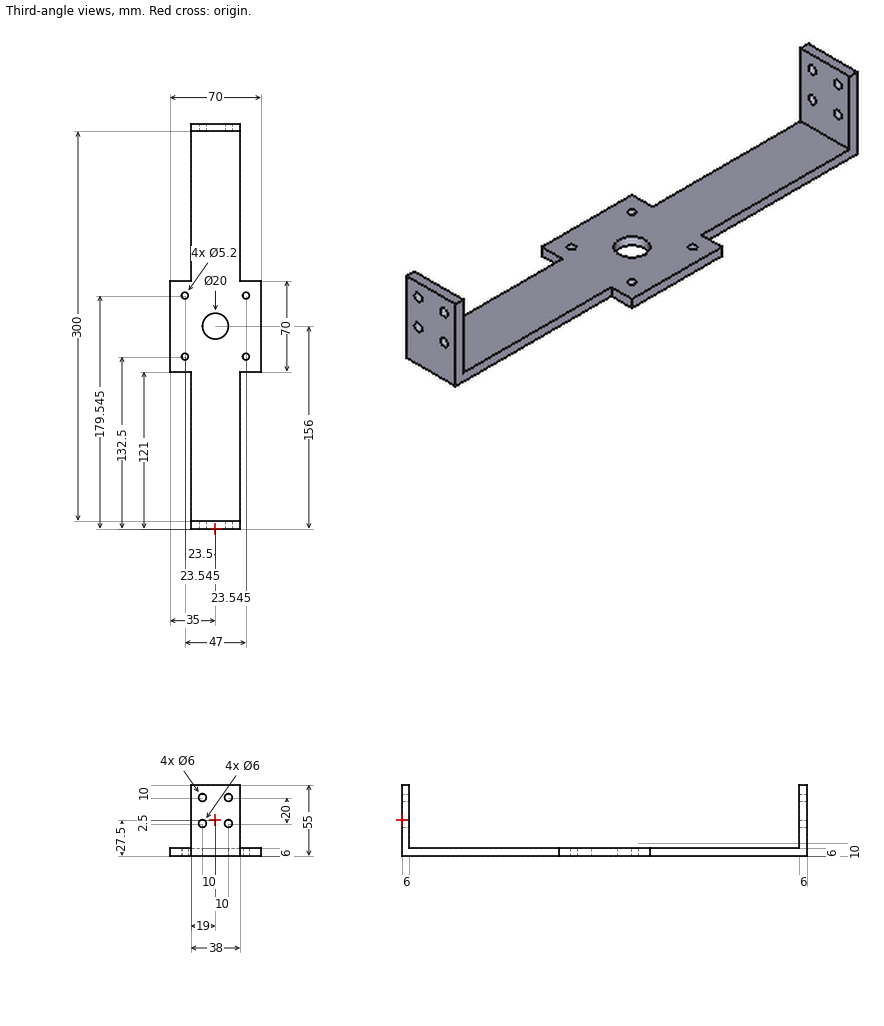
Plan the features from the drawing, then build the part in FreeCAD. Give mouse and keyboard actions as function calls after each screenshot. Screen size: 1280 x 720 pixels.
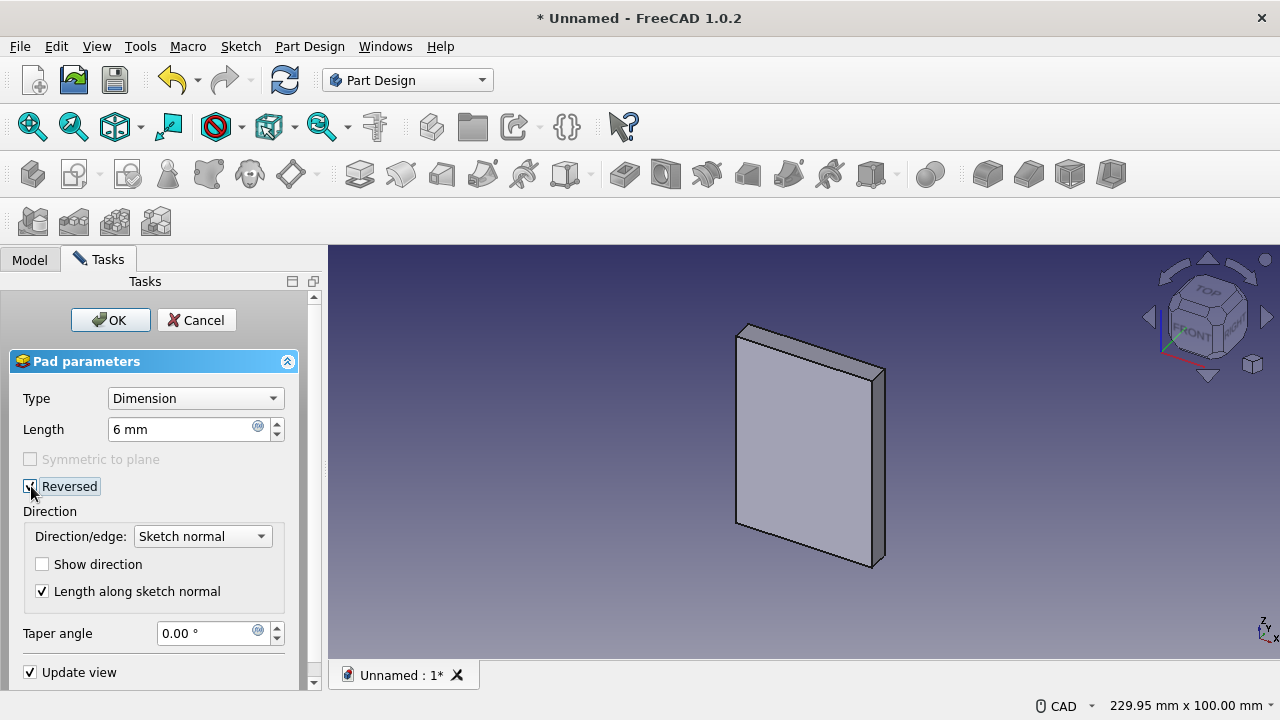
click(111, 320)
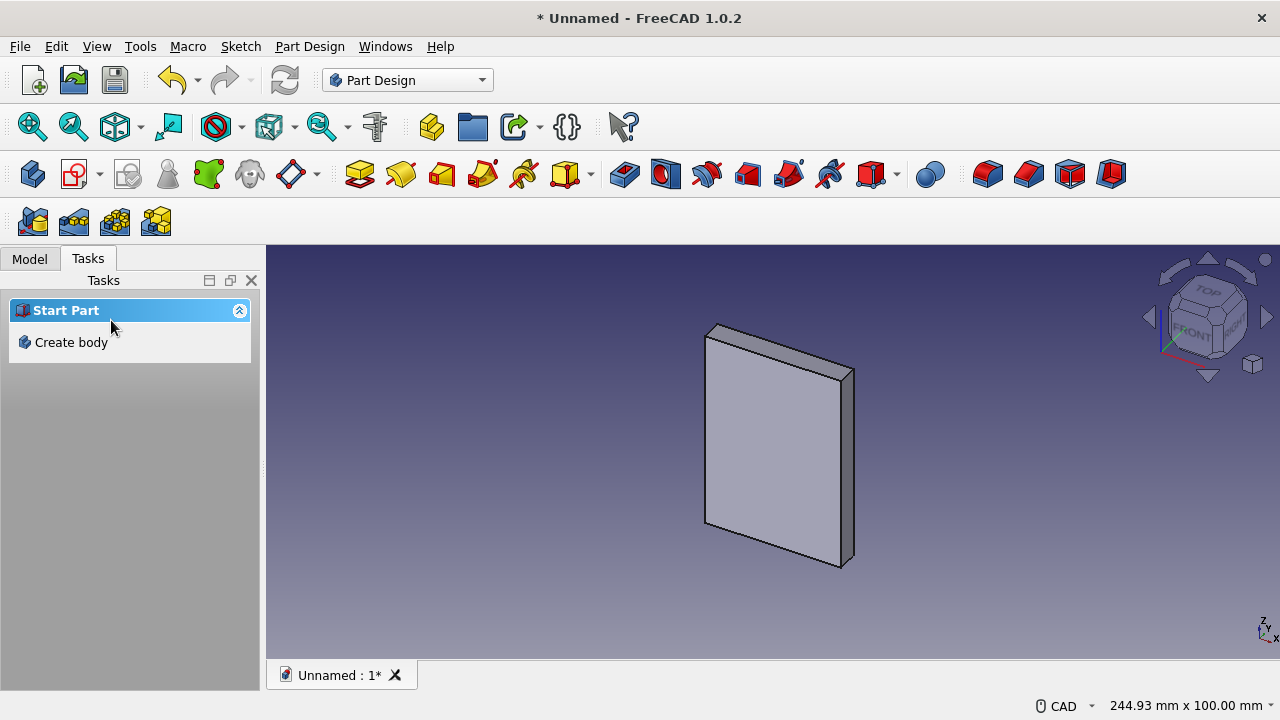
key(4)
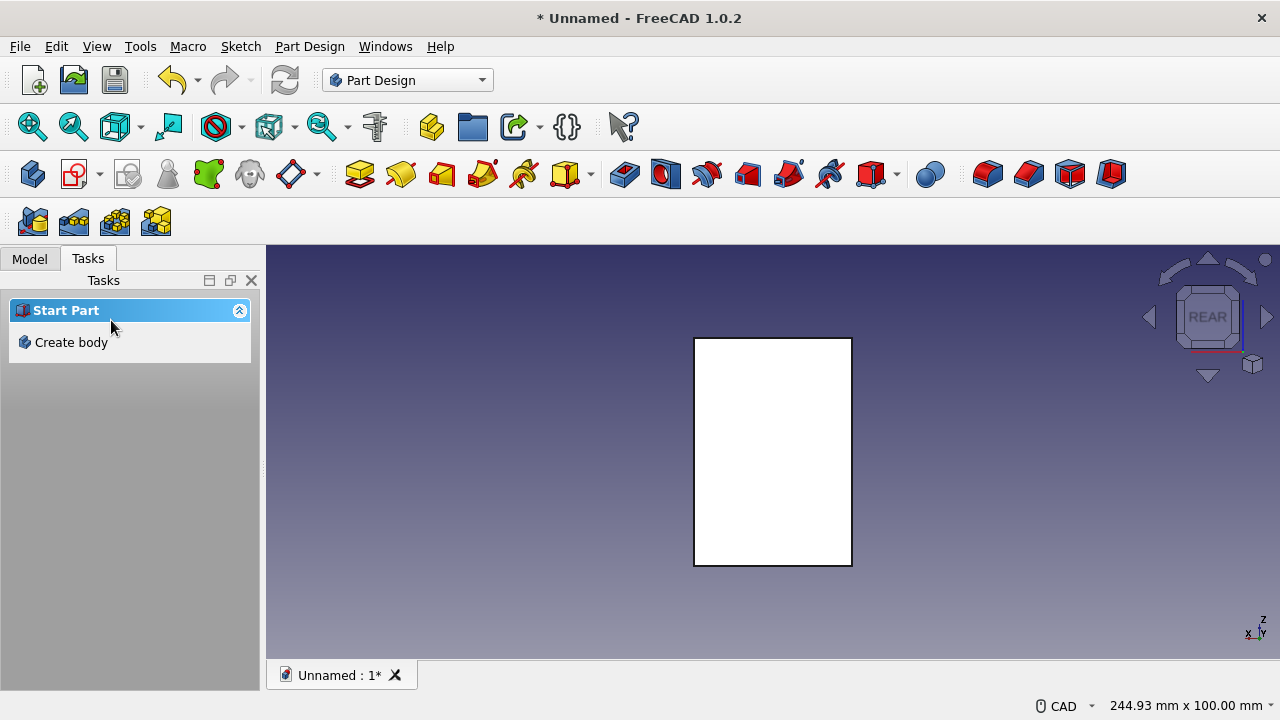
click(773, 418)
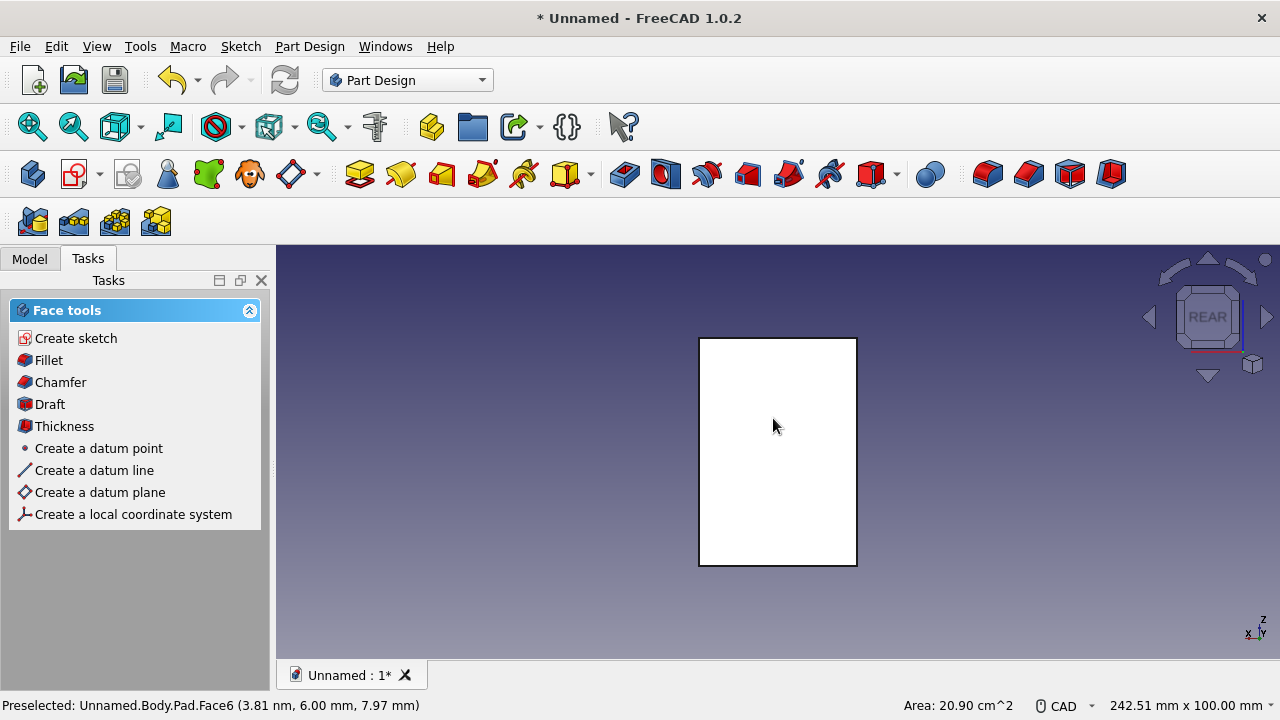
click(74, 174)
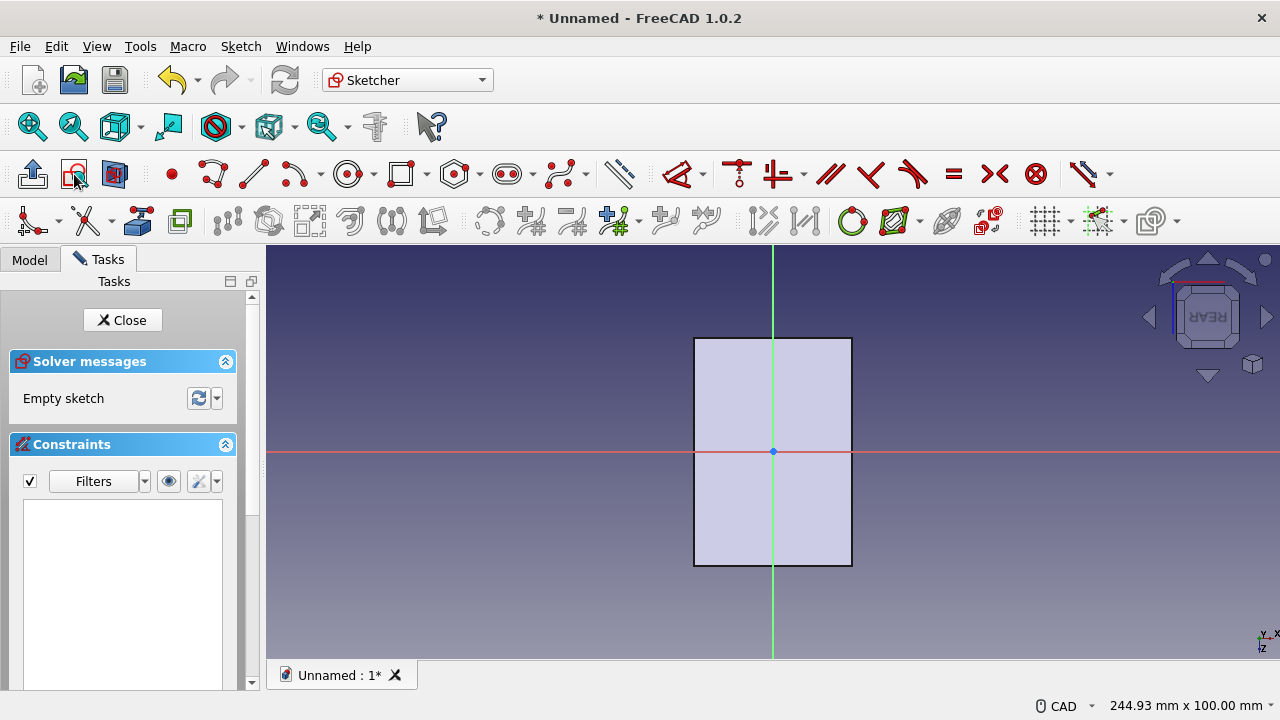
scroll(829, 508, up, 4)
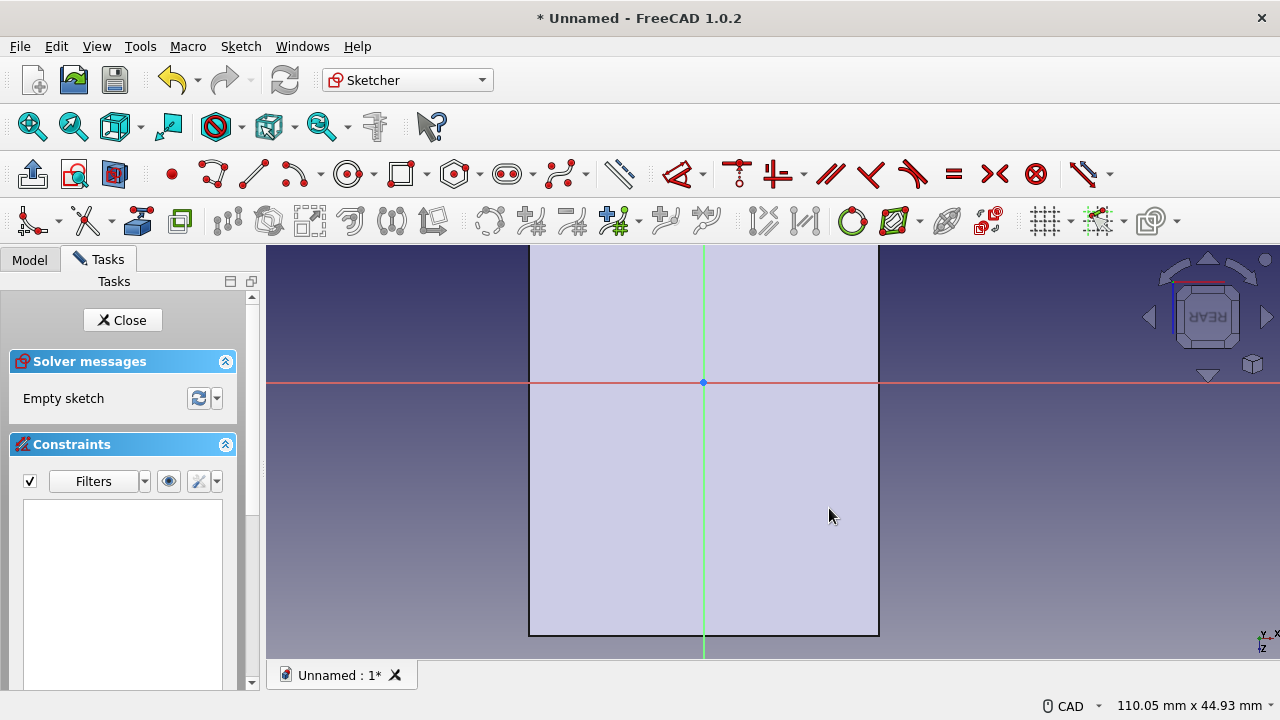
click(348, 174)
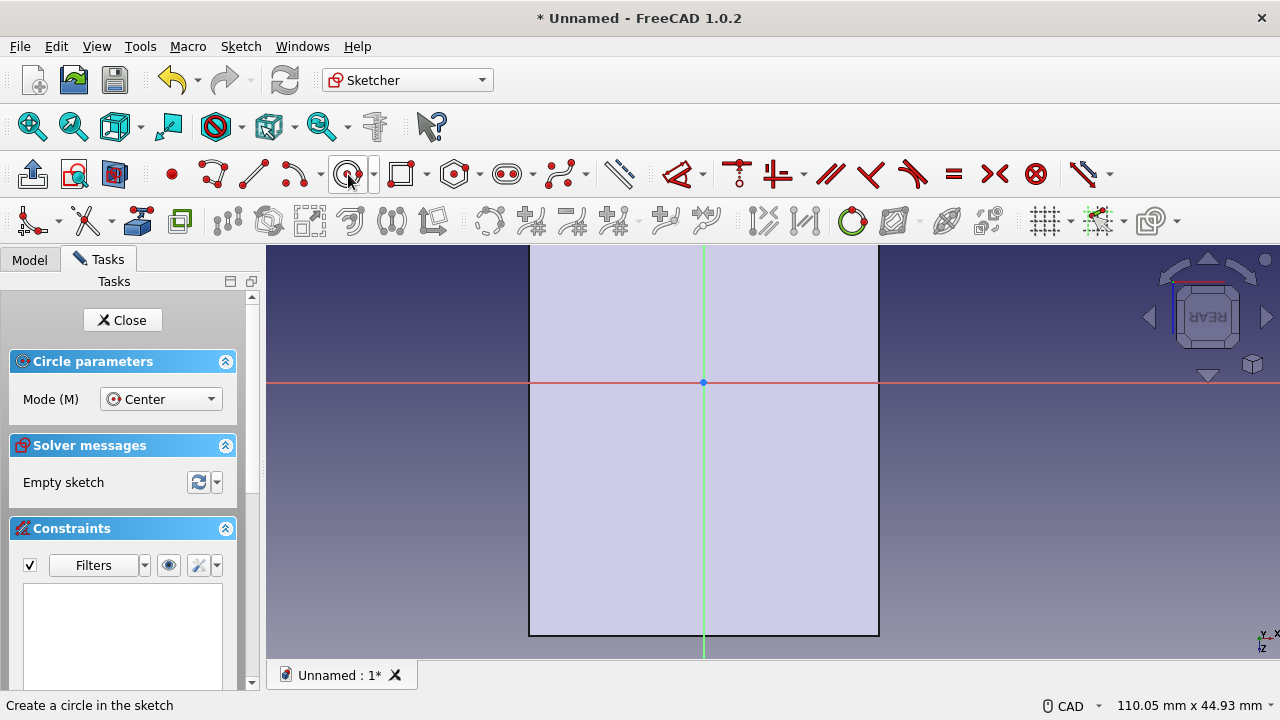
click(612, 360)
move(631, 340)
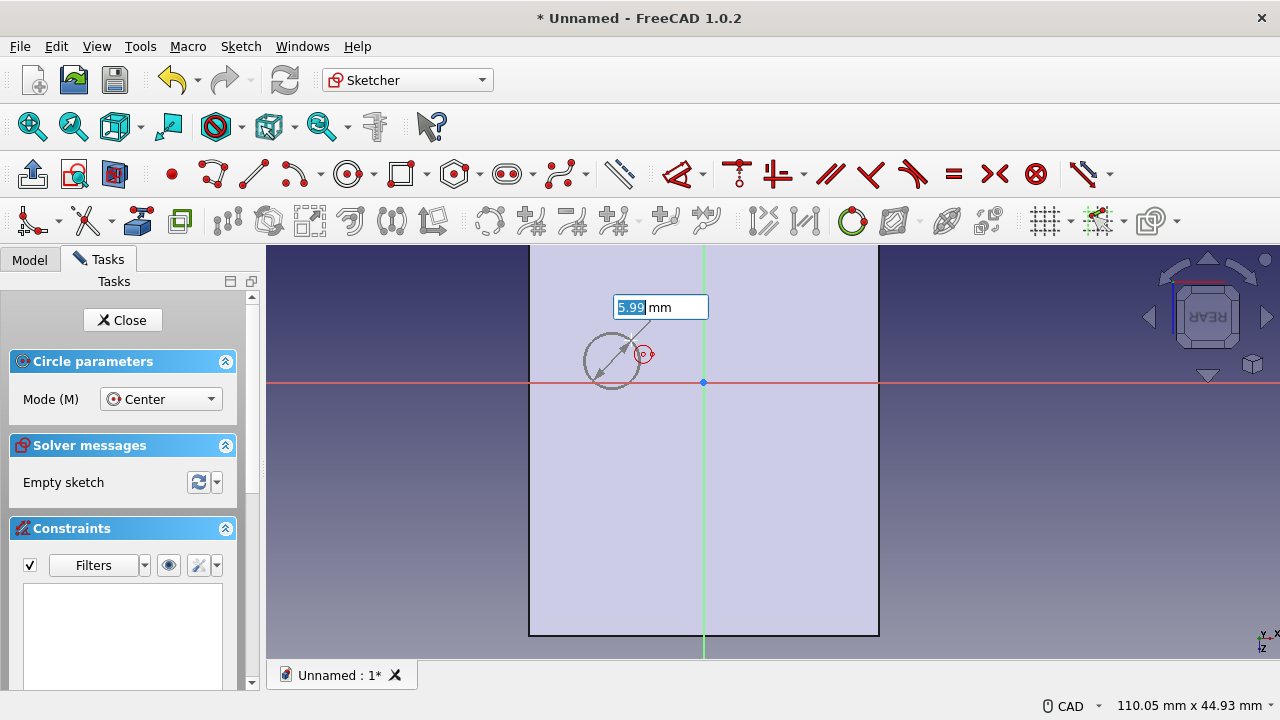
text(6)
key(Return)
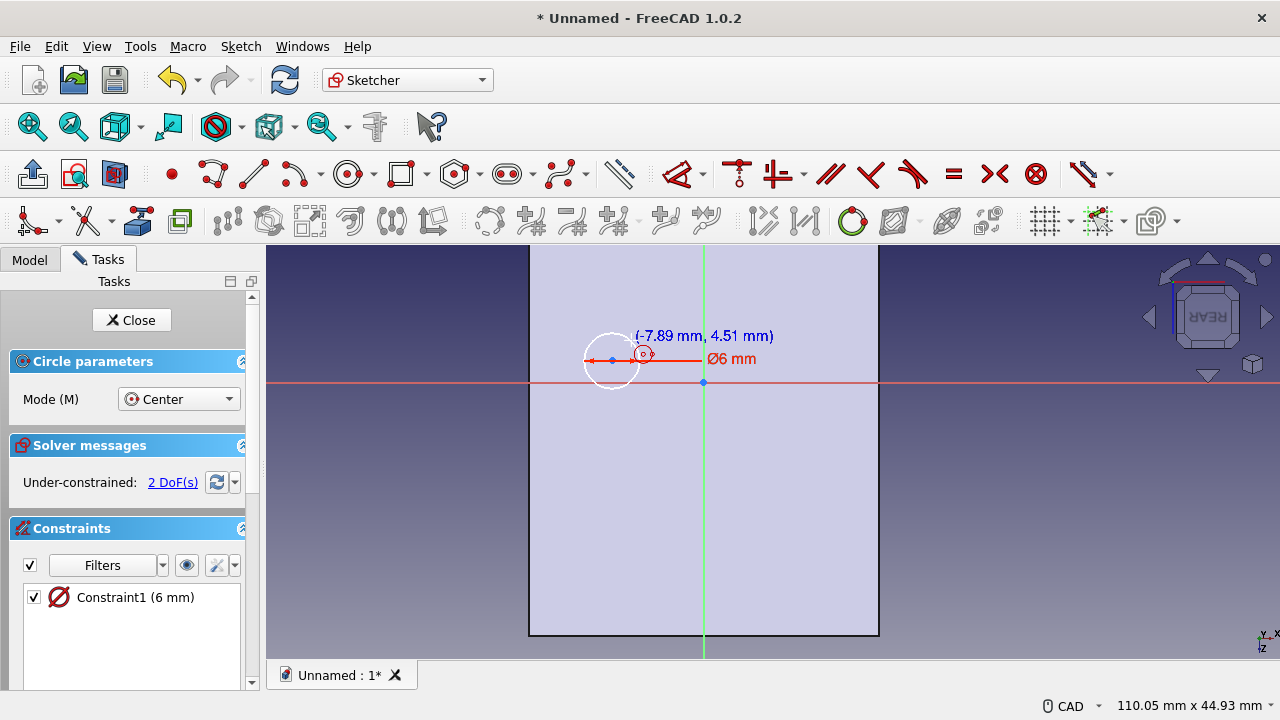
click(796, 360)
move(815, 340)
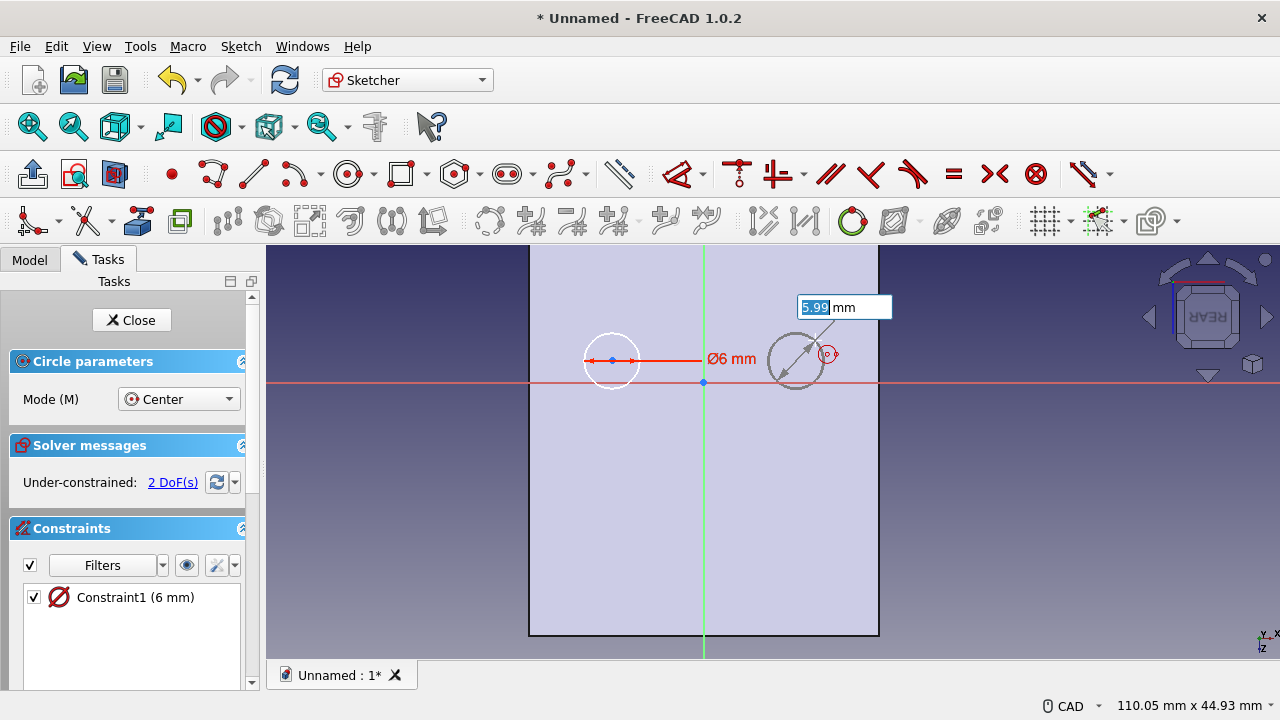
text(6)
key(Return)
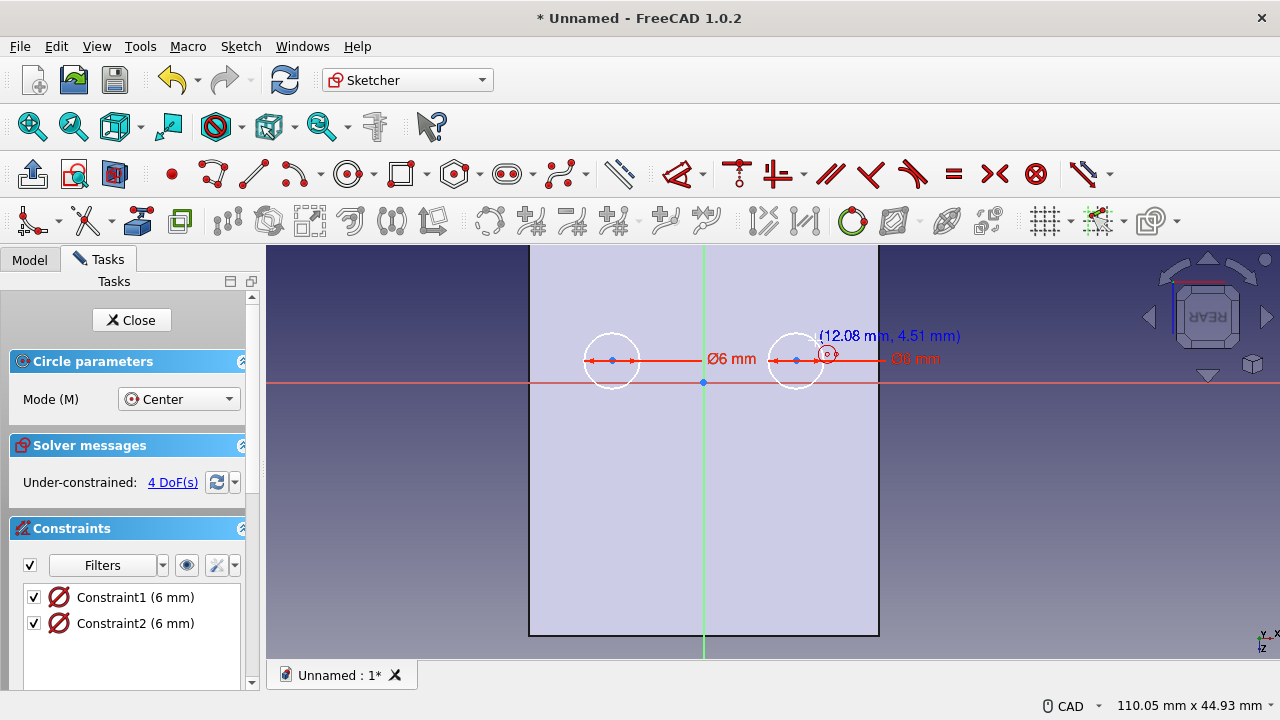
click(796, 544)
move(815, 524)